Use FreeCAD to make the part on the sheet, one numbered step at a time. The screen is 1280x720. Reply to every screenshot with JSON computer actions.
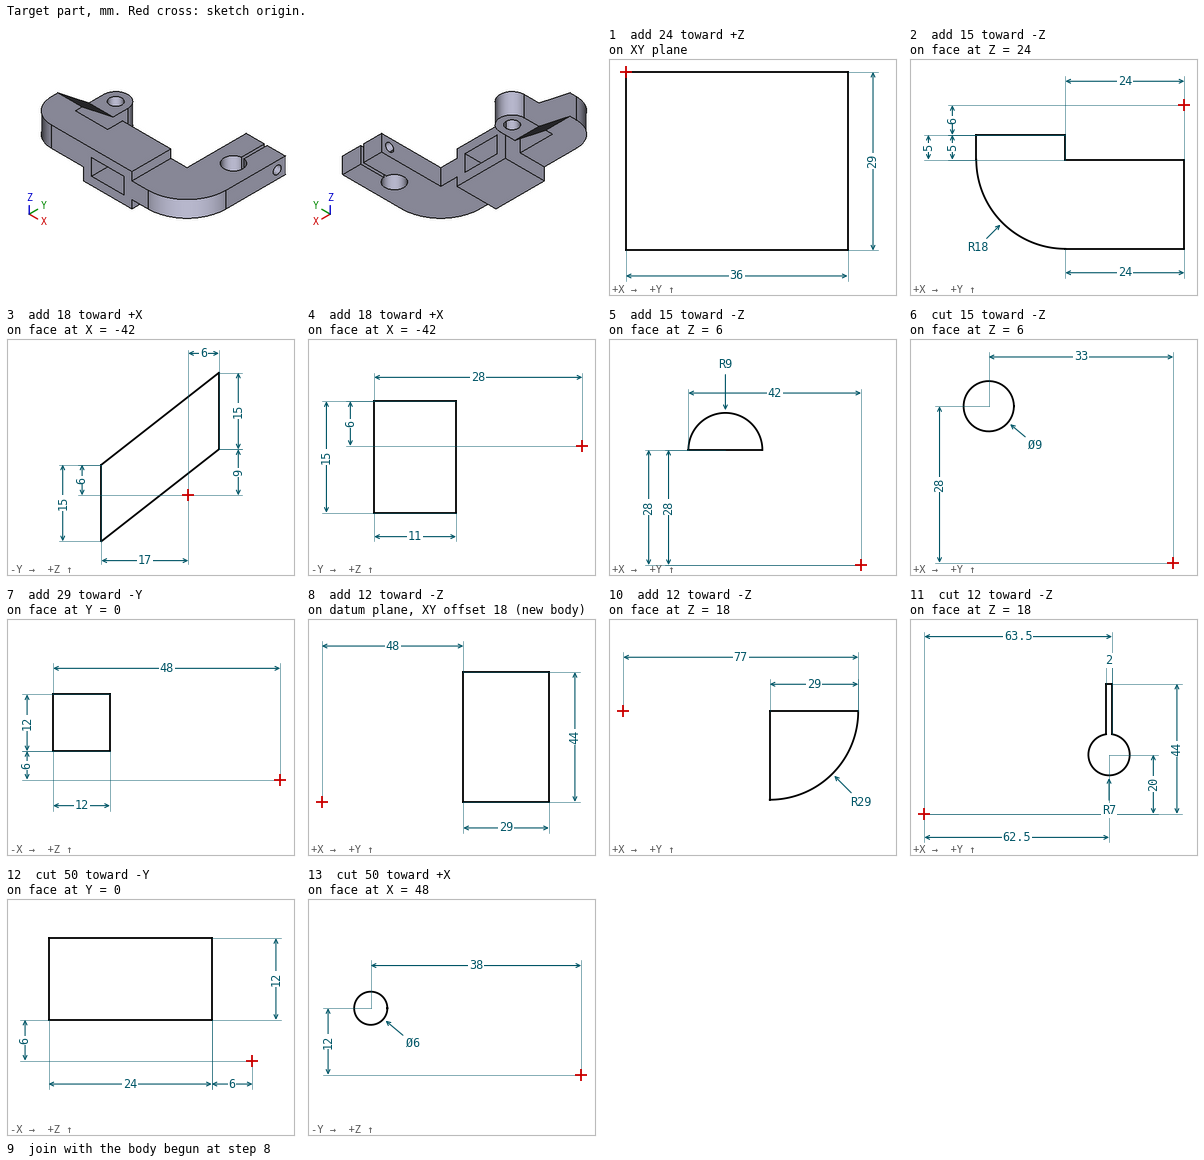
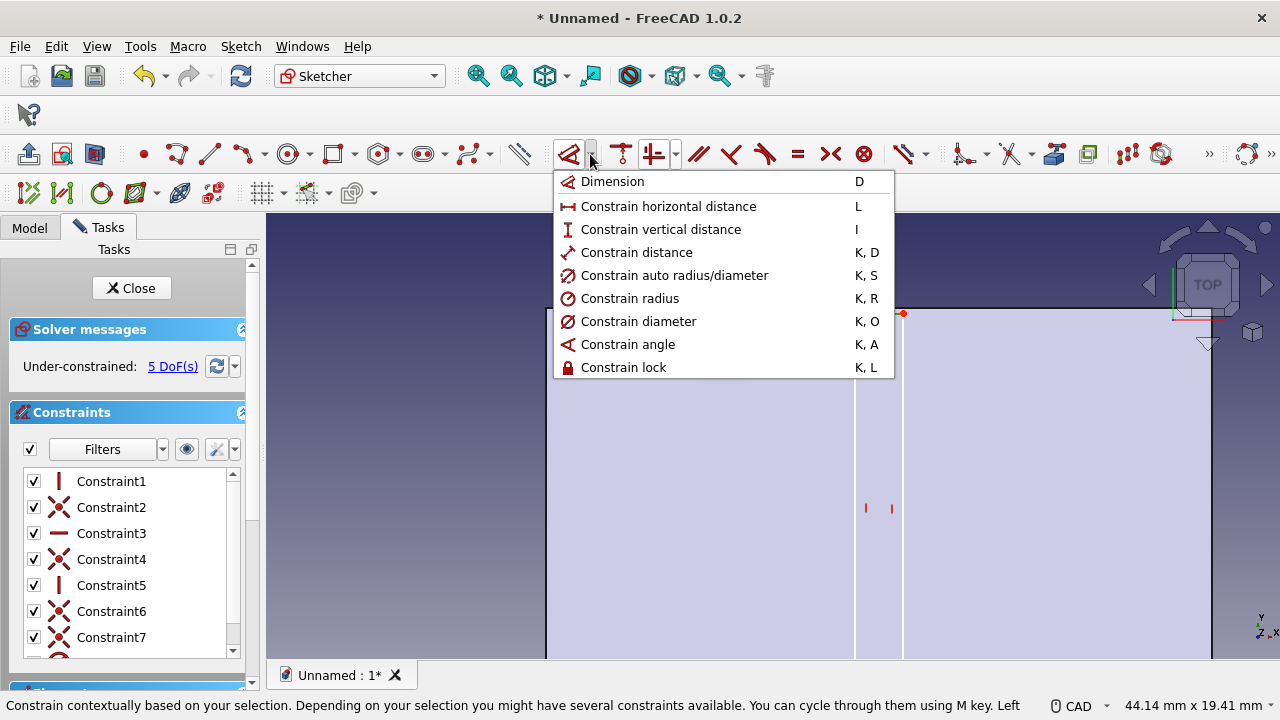
{"action": "left_click", "coordinate": [724, 206]}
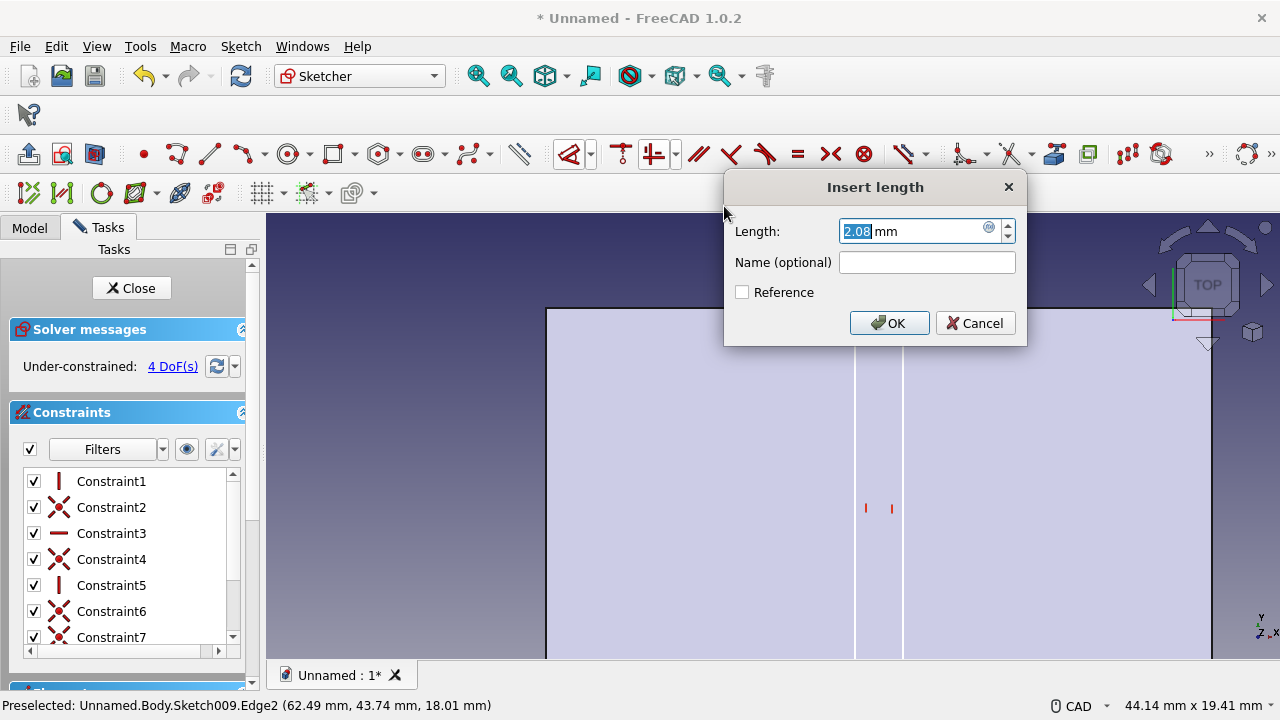
{"action": "type", "text": "2"}
{"action": "key", "text": "Return"}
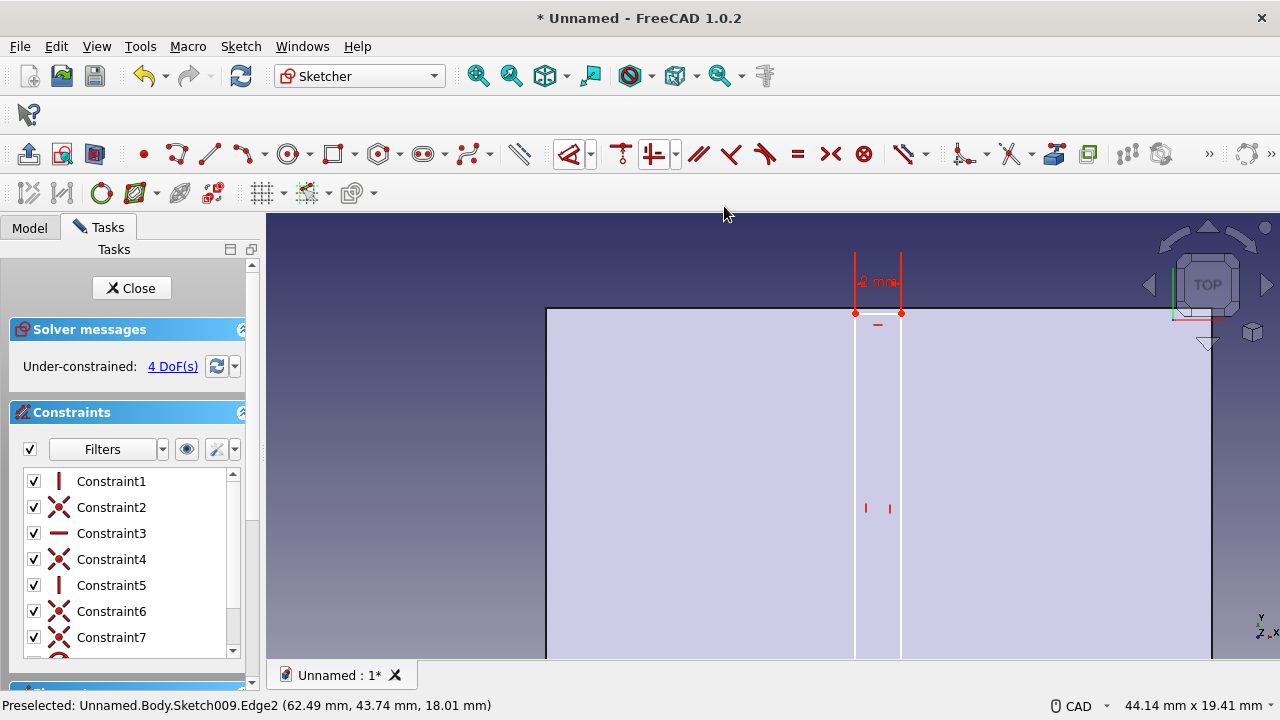
{"action": "scroll", "coordinate": [879, 313], "scroll_direction": "down", "scroll_amount": 7}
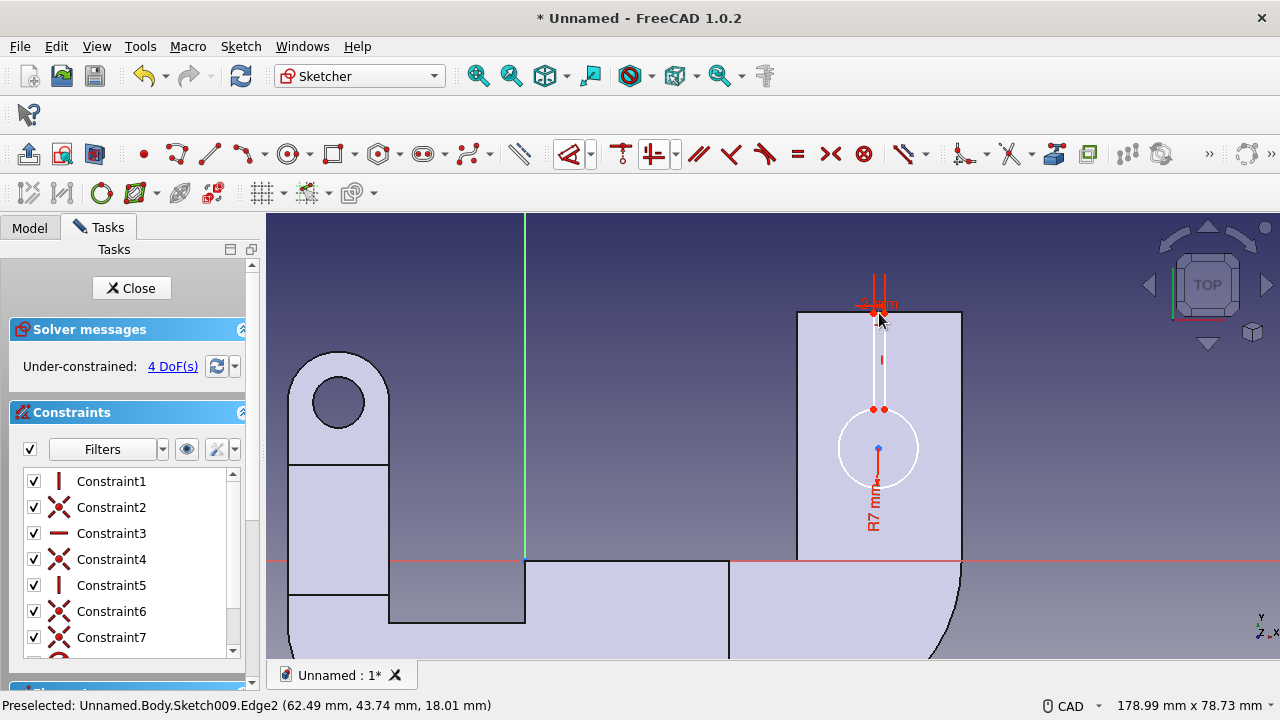
{"action": "left_click", "coordinate": [885, 313]}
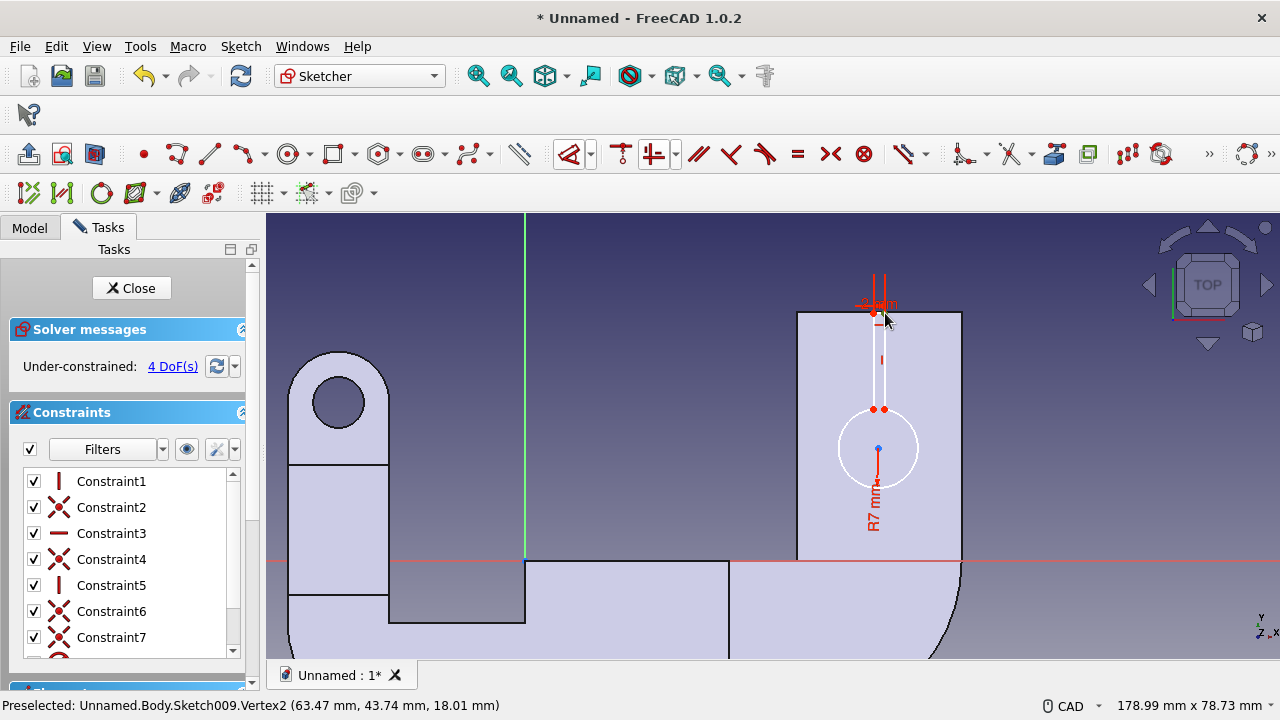
{"action": "left_click", "coordinate": [590, 154]}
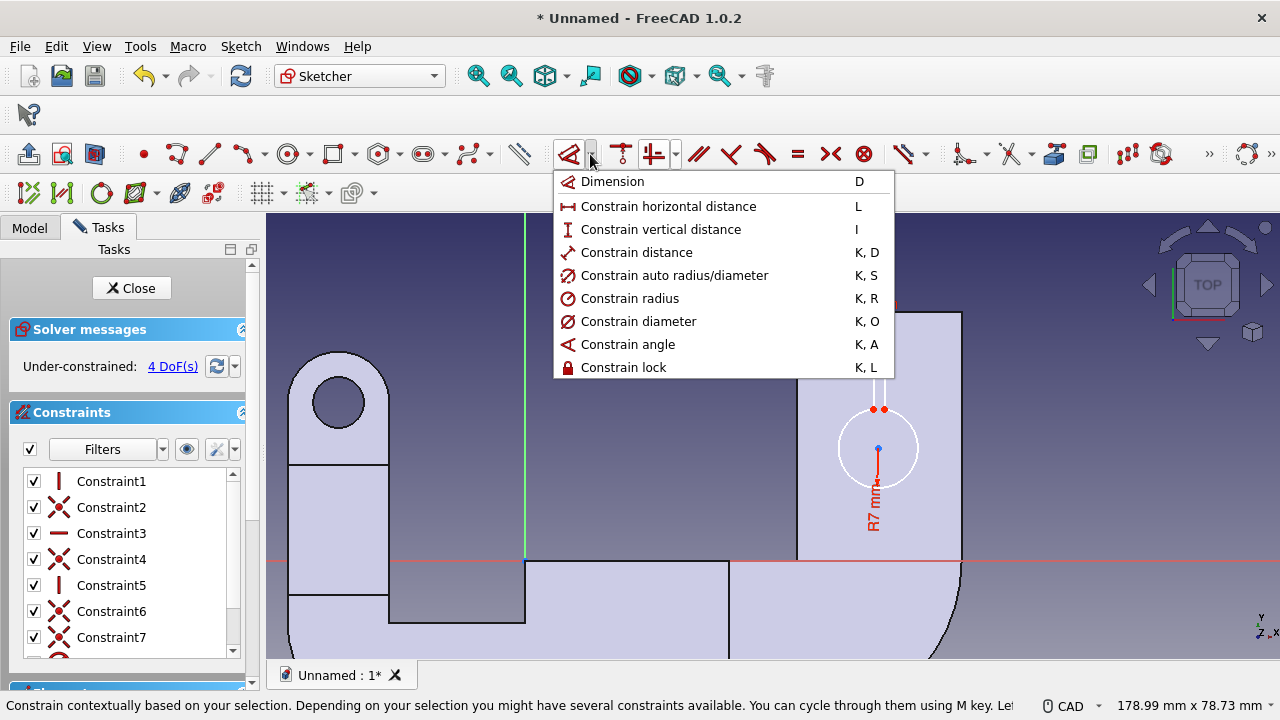
{"action": "left_click", "coordinate": [724, 230]}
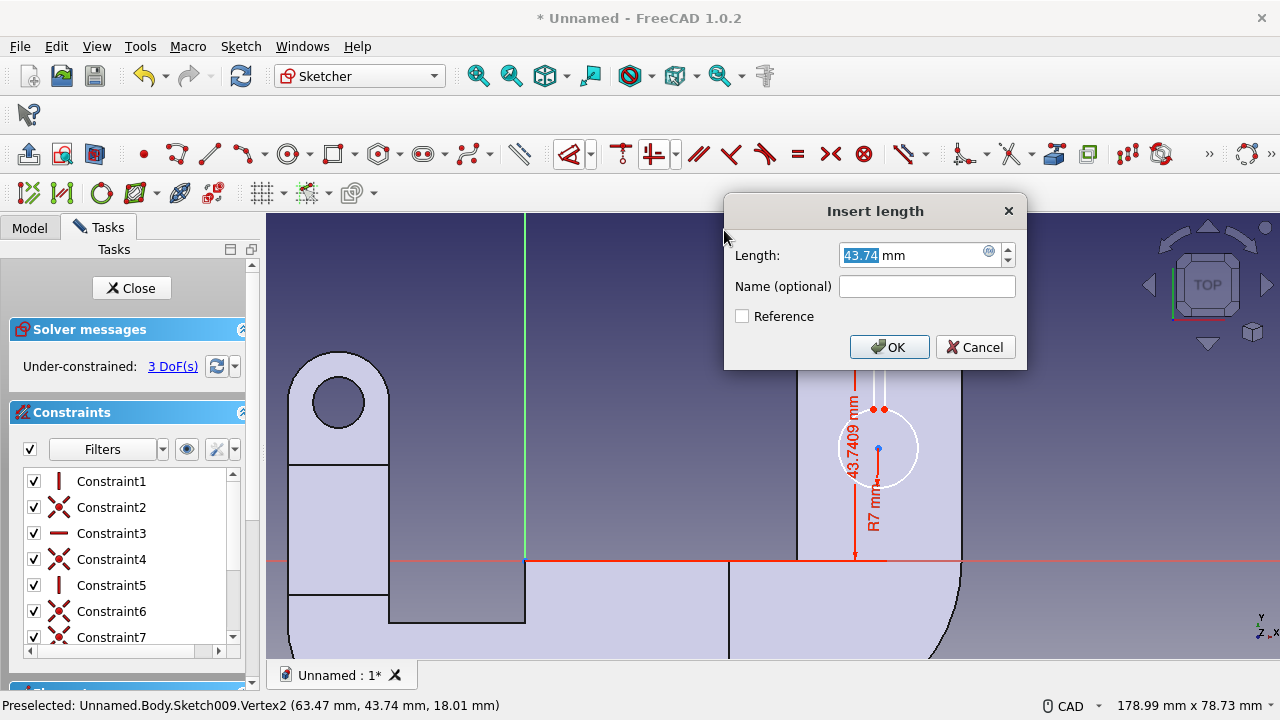
{"action": "type", "text": "44"}
{"action": "key", "text": "Return"}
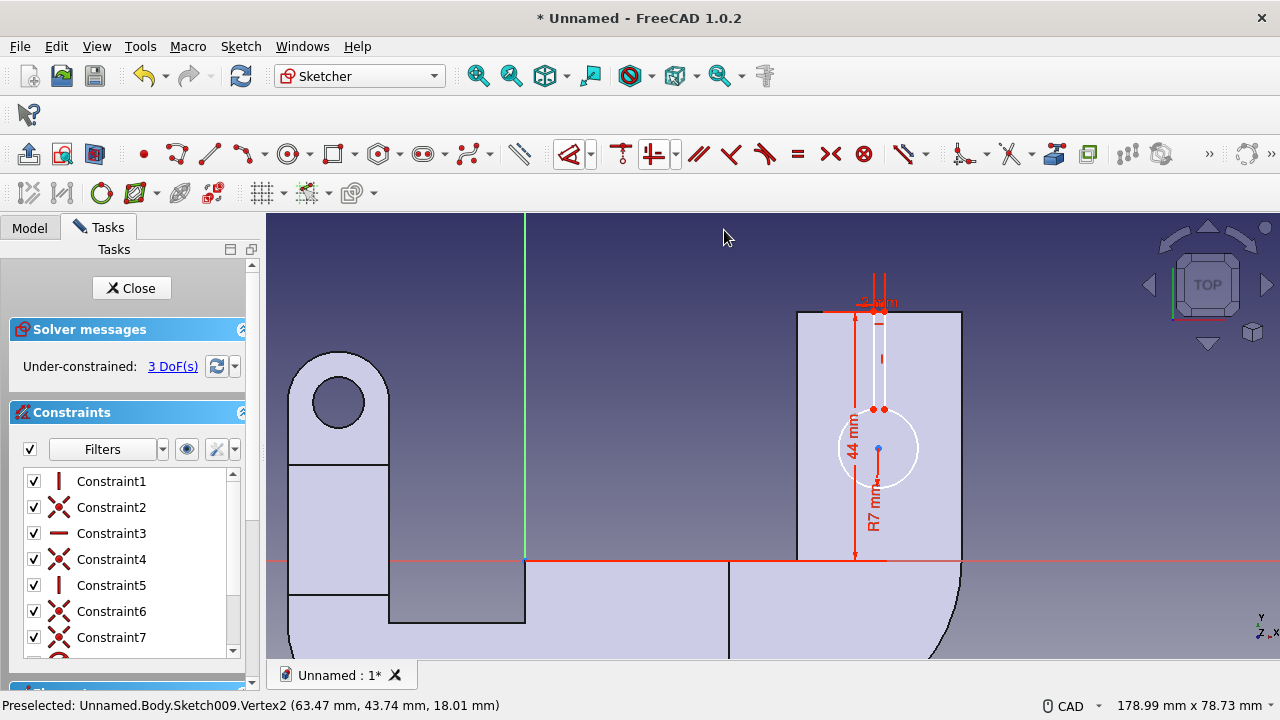
{"action": "left_click", "coordinate": [878, 448]}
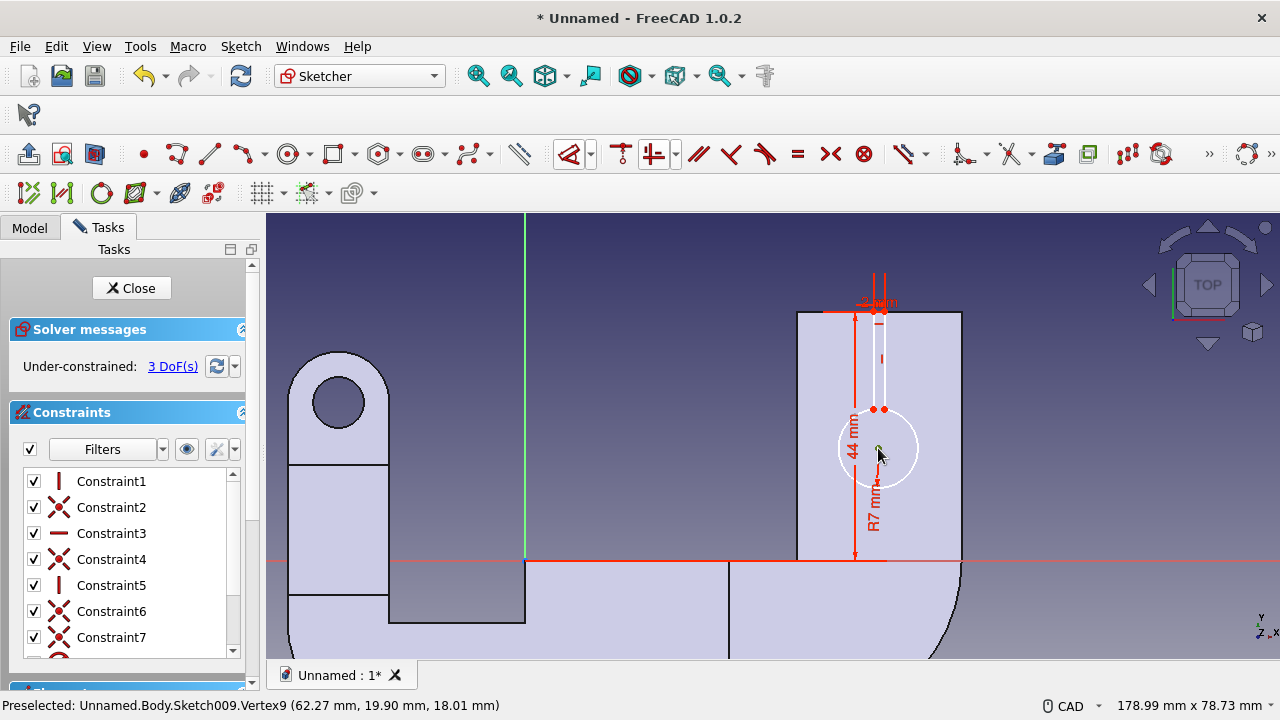
{"action": "key", "text": "i"}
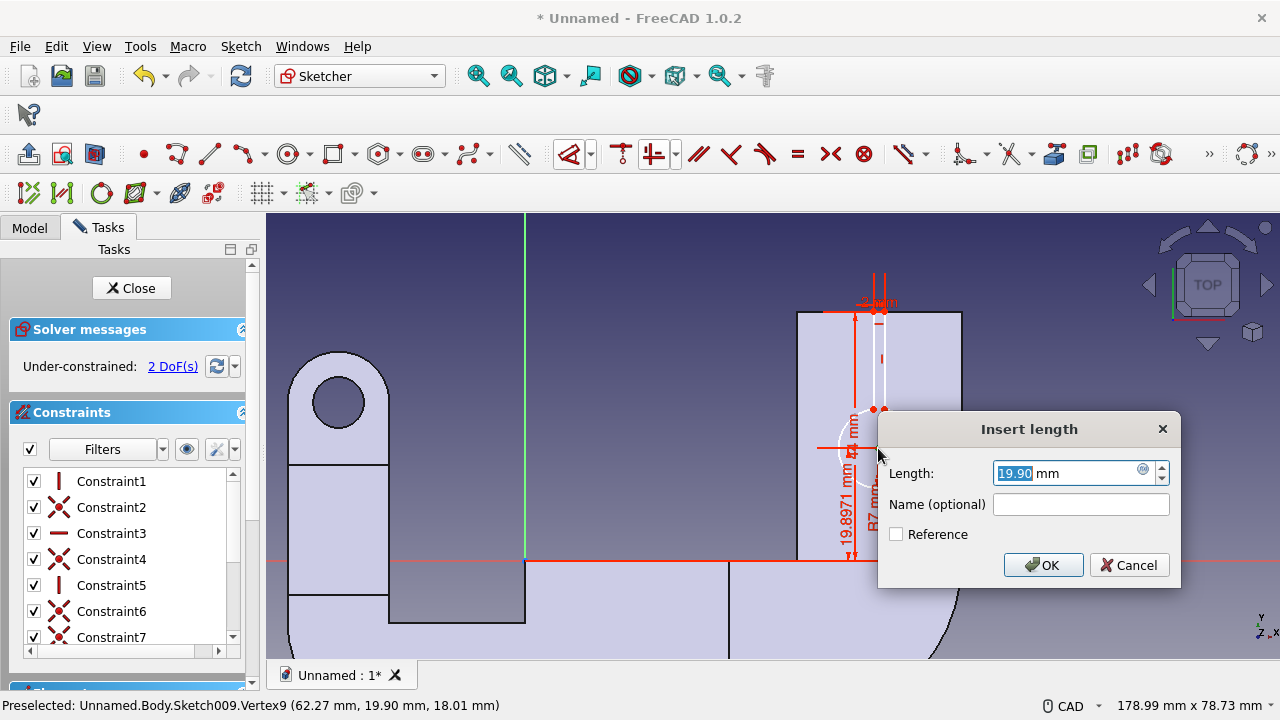
{"action": "type", "text": "20"}
{"action": "key", "text": "Return"}